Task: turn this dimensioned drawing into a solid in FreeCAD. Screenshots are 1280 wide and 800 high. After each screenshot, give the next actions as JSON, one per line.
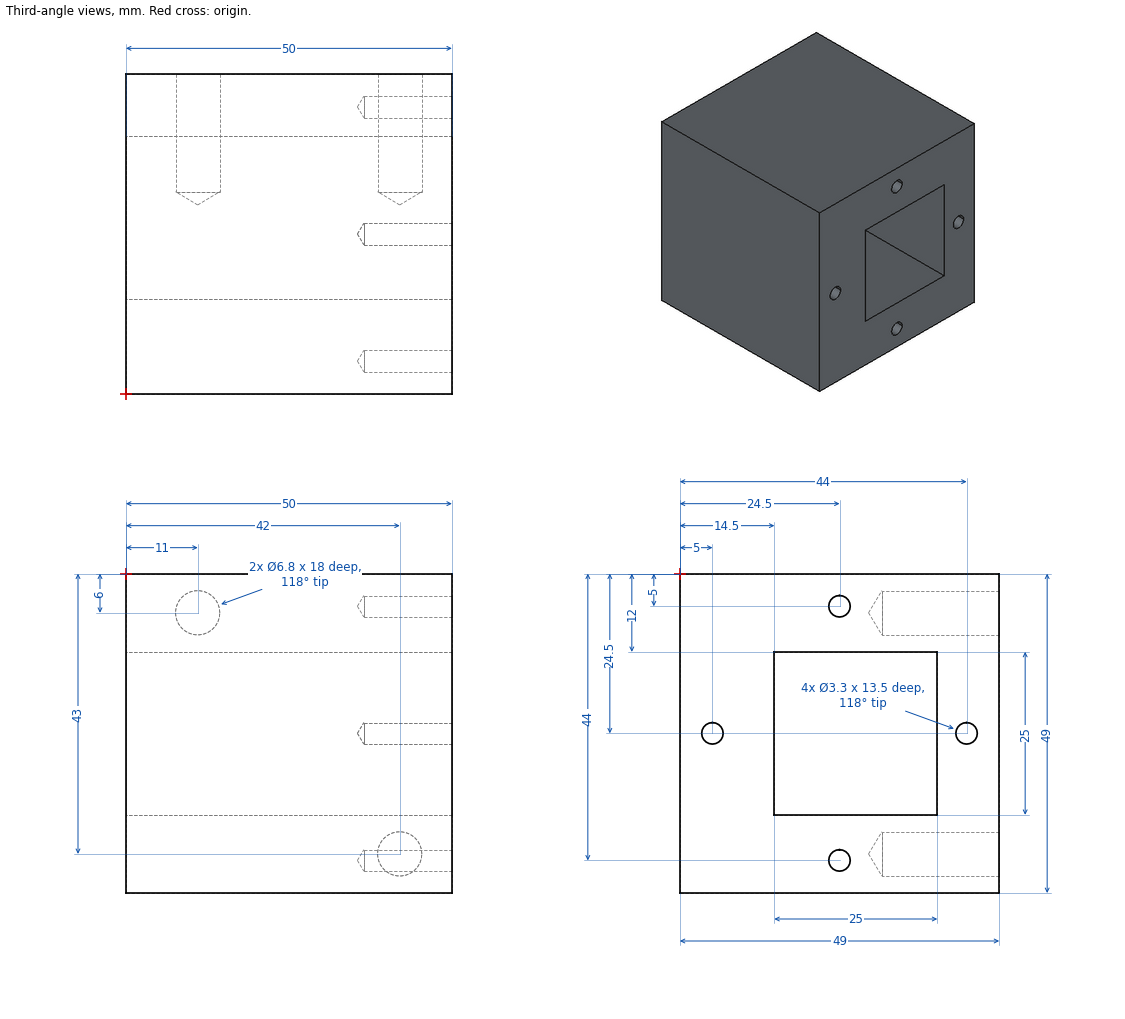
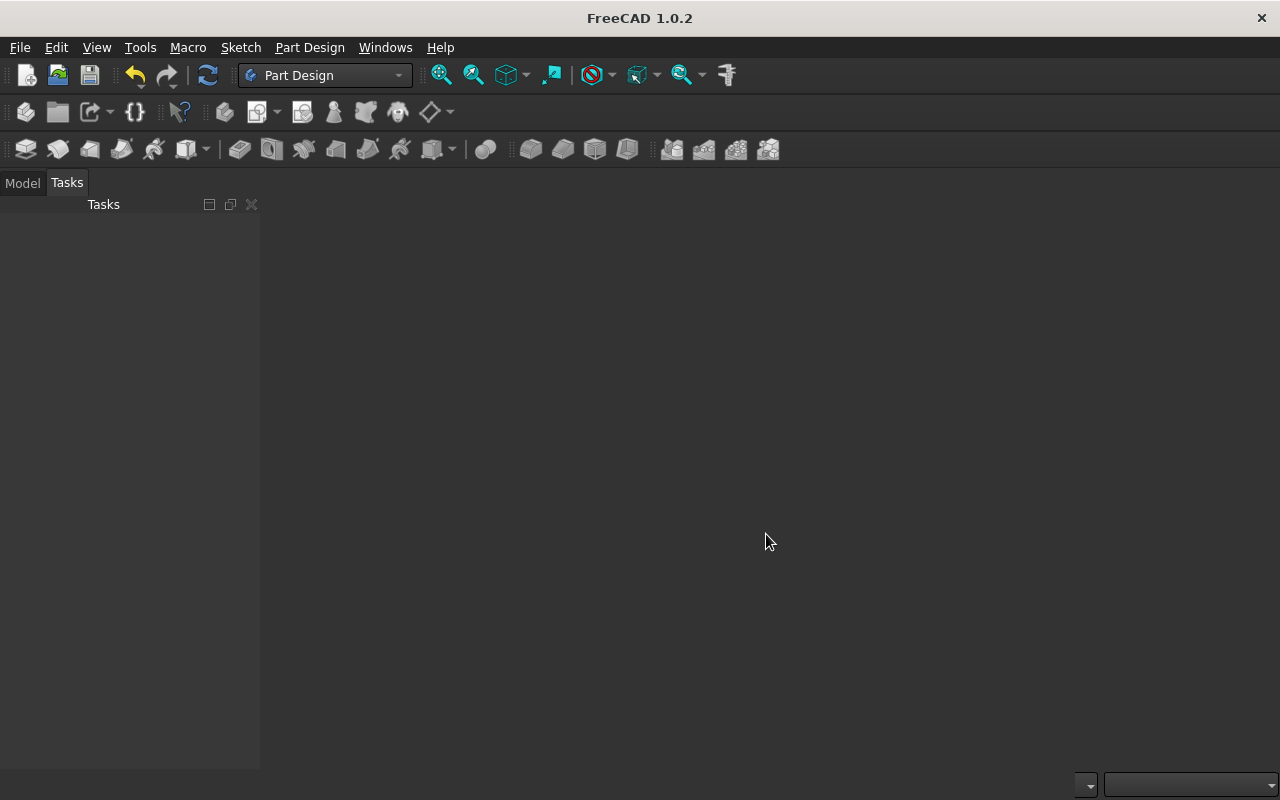
{"action": "key", "text": "ctrl+n"}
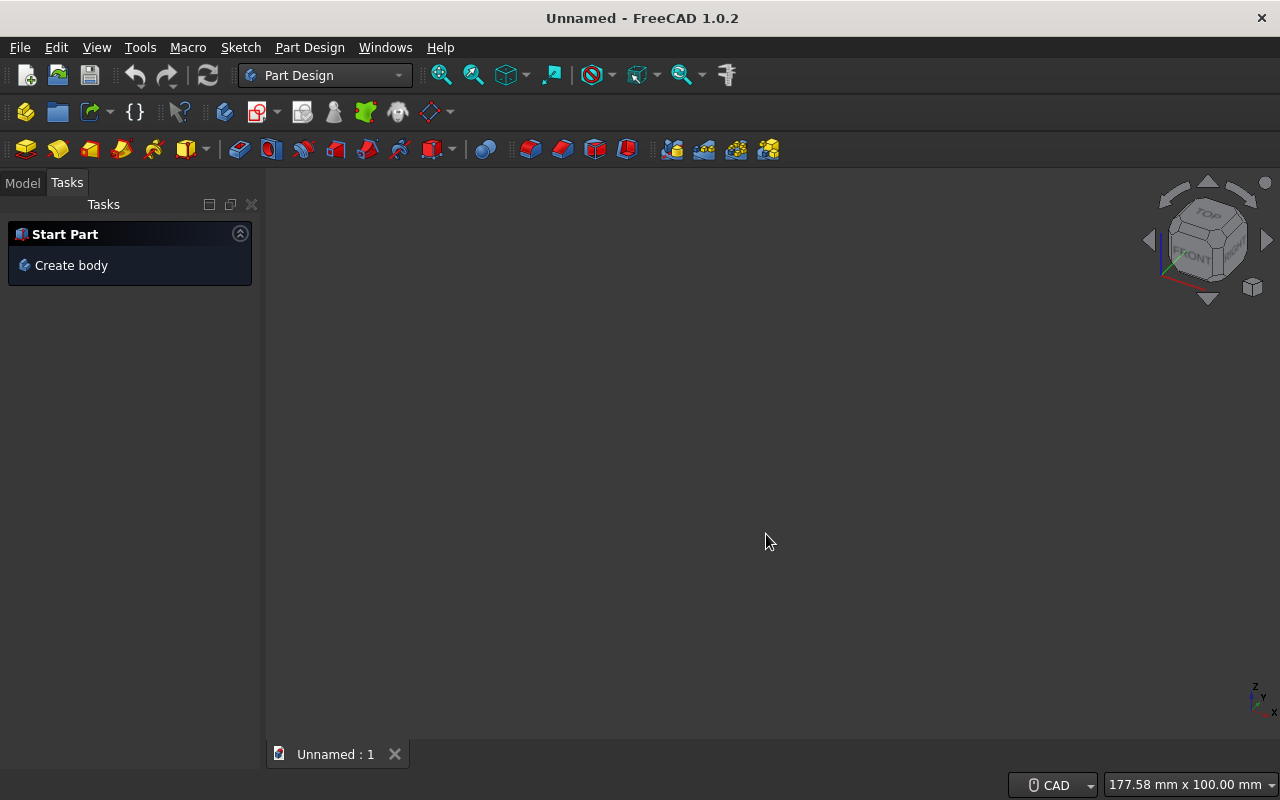
{"action": "left_click", "coordinate": [258, 112]}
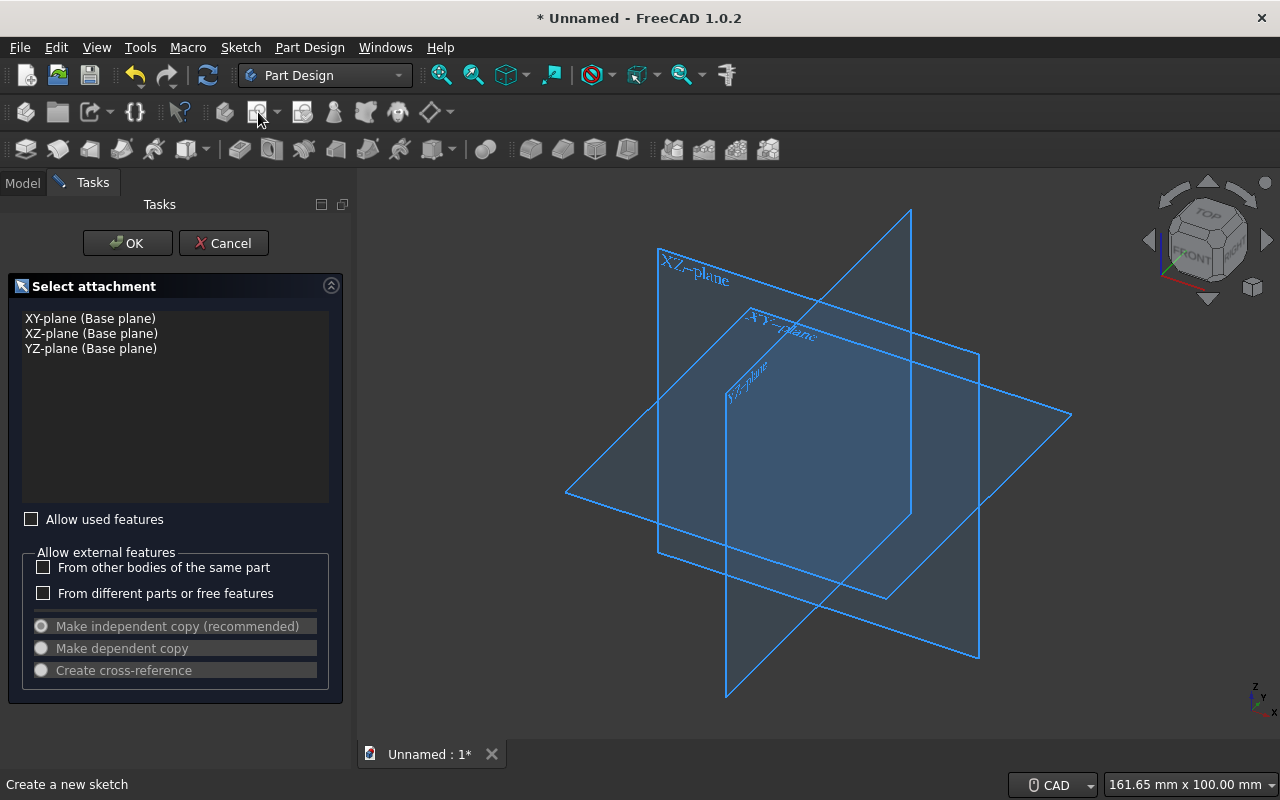
{"action": "left_click", "coordinate": [82, 348]}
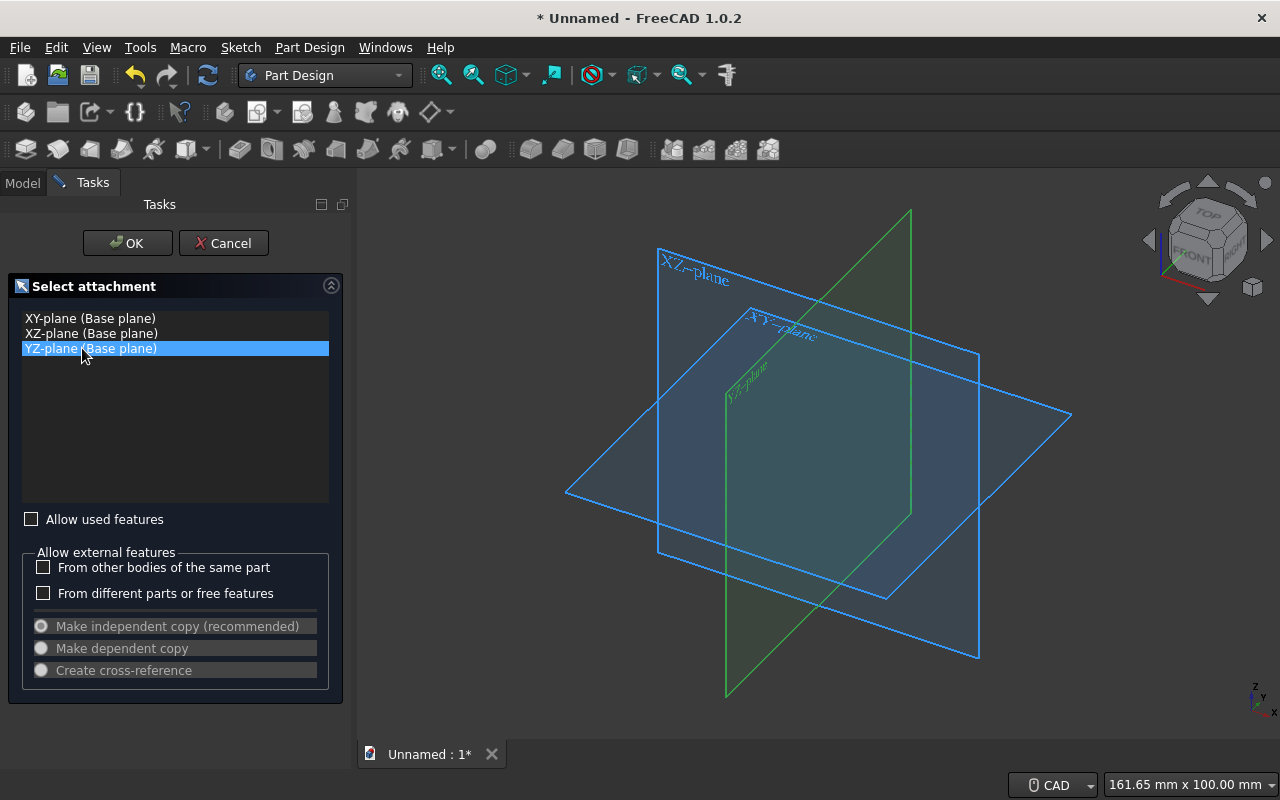
{"action": "left_click", "coordinate": [128, 243]}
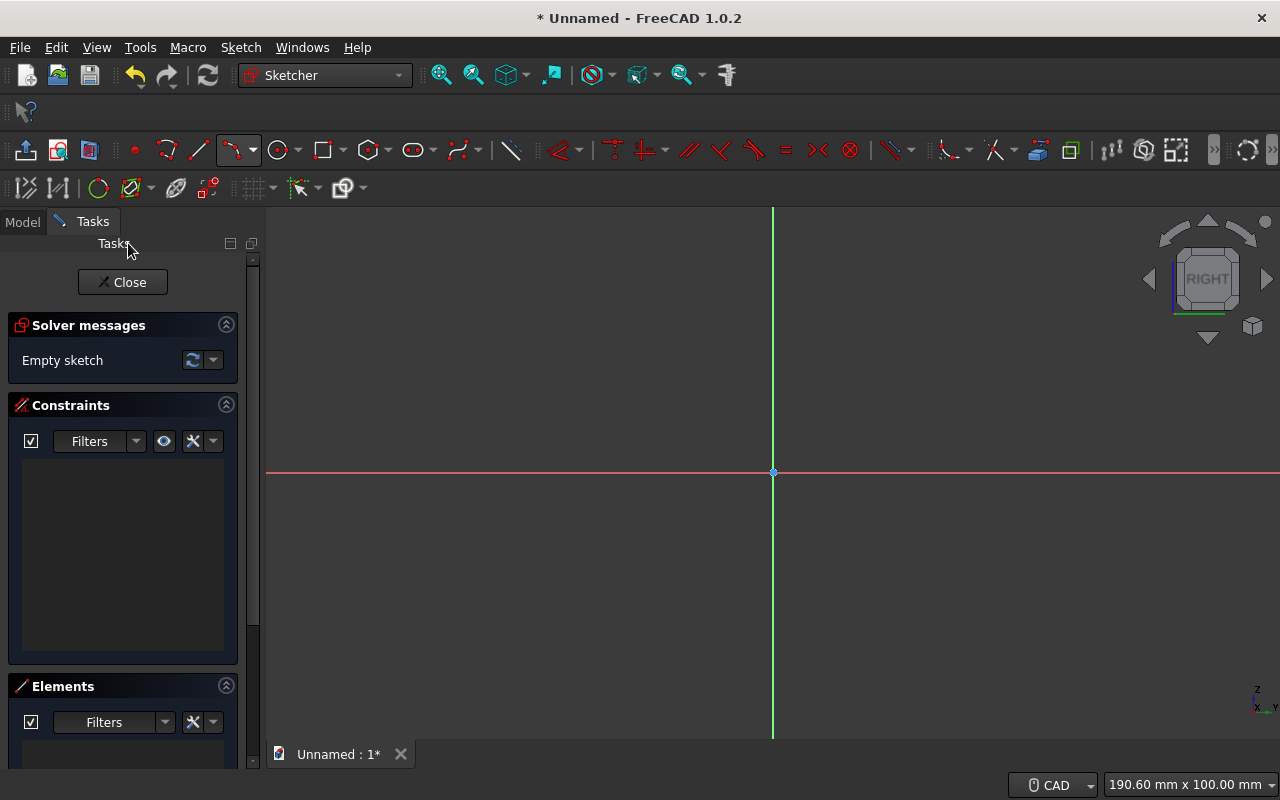
{"action": "scroll", "coordinate": [294, 235], "scroll_direction": "down", "scroll_amount": 1}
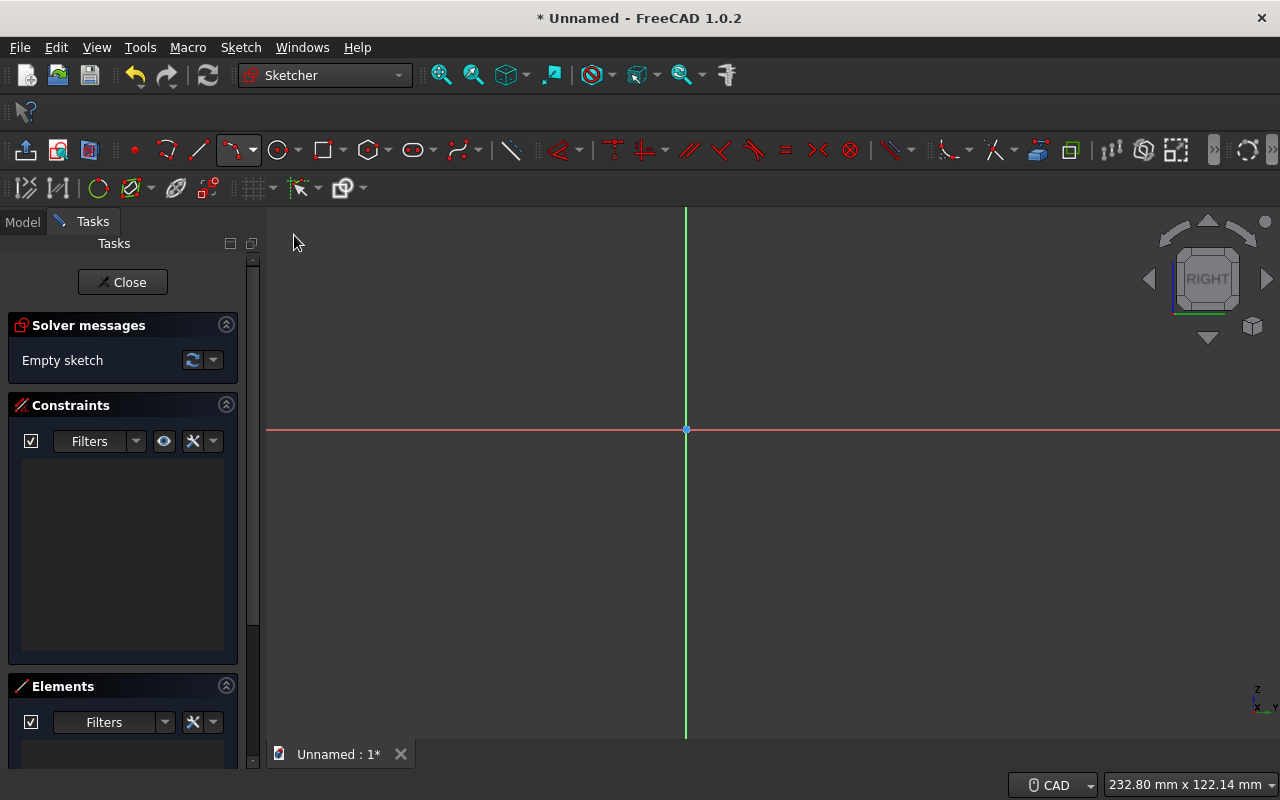
{"action": "scroll", "coordinate": [973, 666], "scroll_direction": "up", "scroll_amount": 2}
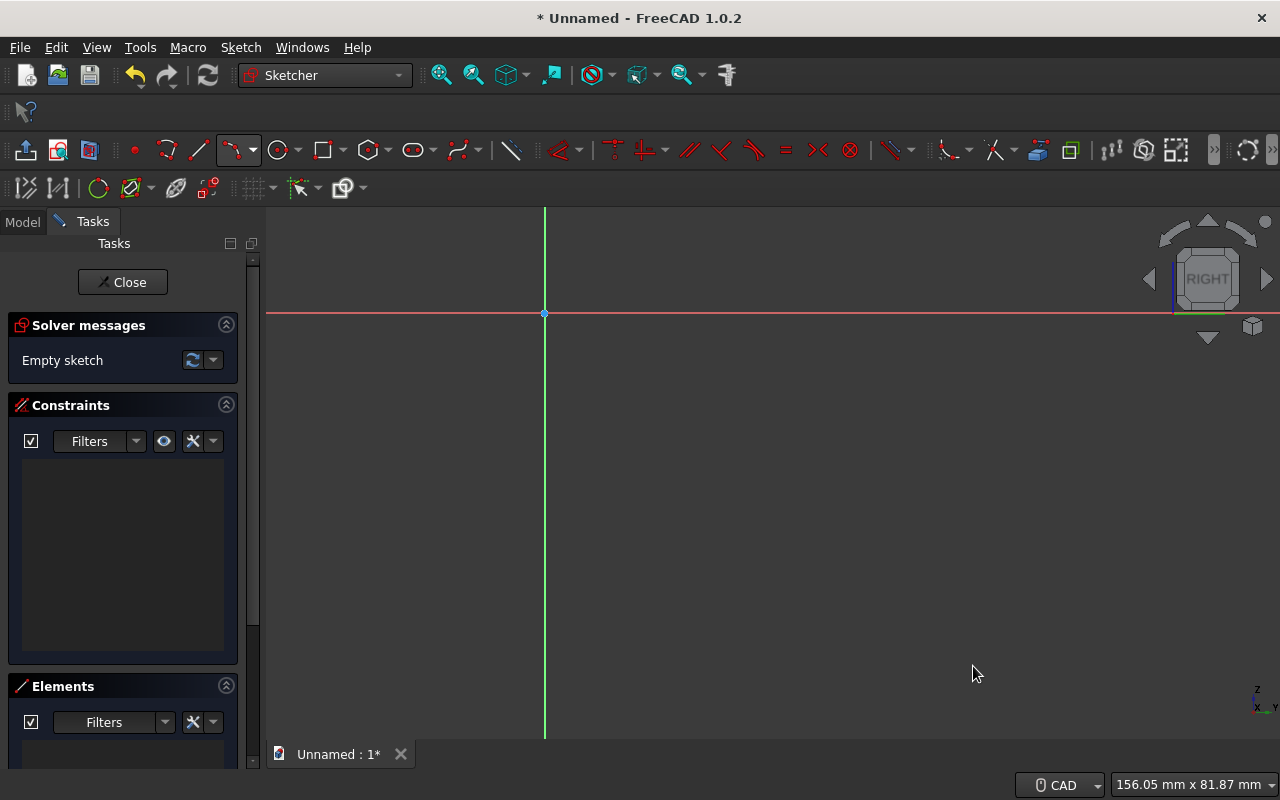
{"action": "key", "text": "g r"}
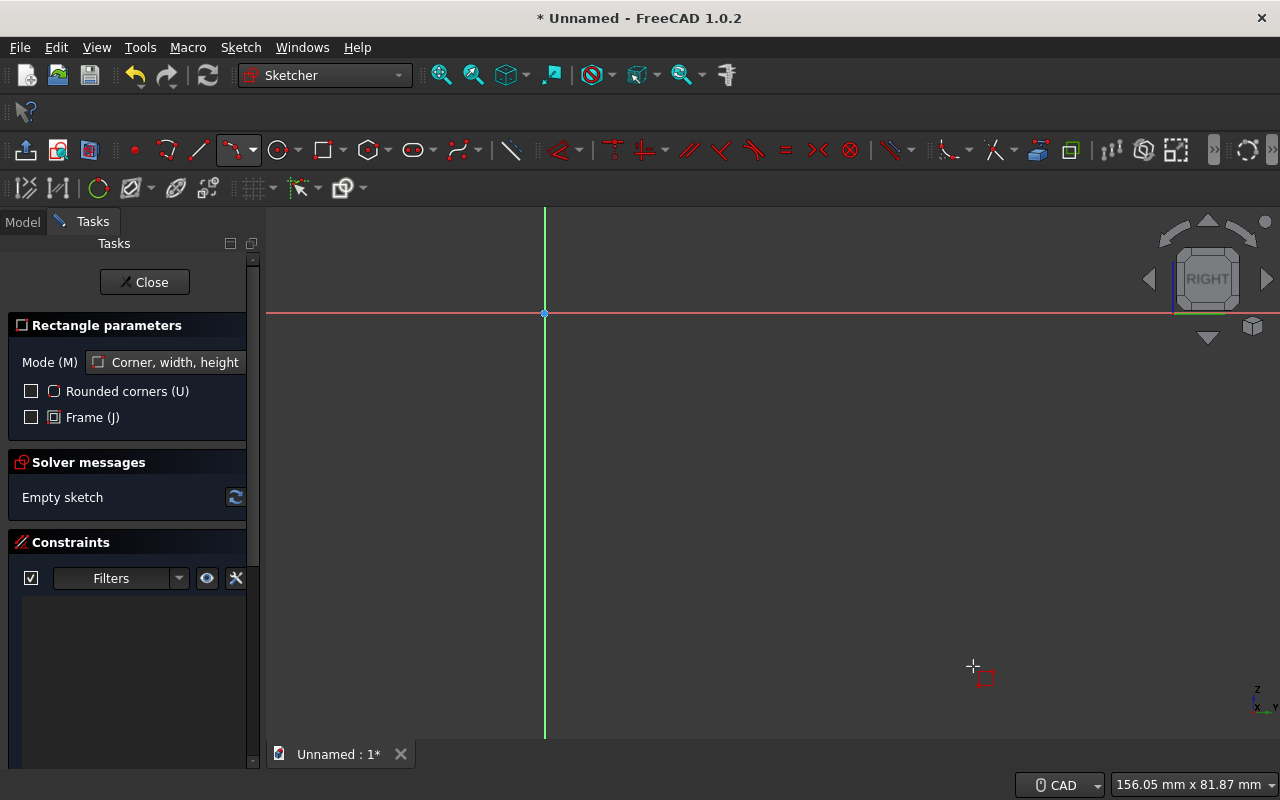
{"action": "left_click", "coordinate": [545, 313]}
{"action": "mouse_move", "coordinate": [863, 632]}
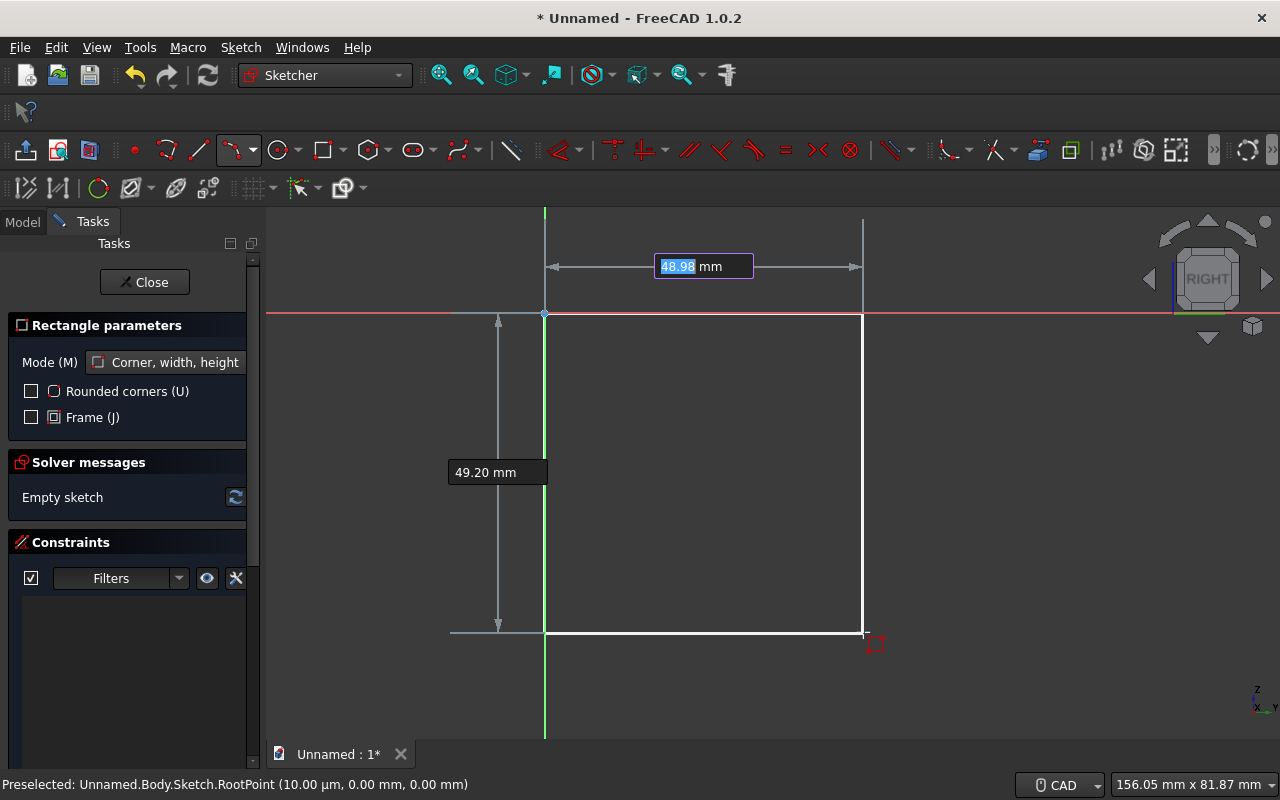
{"action": "type", "text": "49"}
{"action": "key", "text": "Tab"}
{"action": "type", "text": "49"}
{"action": "key", "text": "Return"}
{"action": "key", "text": "Escape"}